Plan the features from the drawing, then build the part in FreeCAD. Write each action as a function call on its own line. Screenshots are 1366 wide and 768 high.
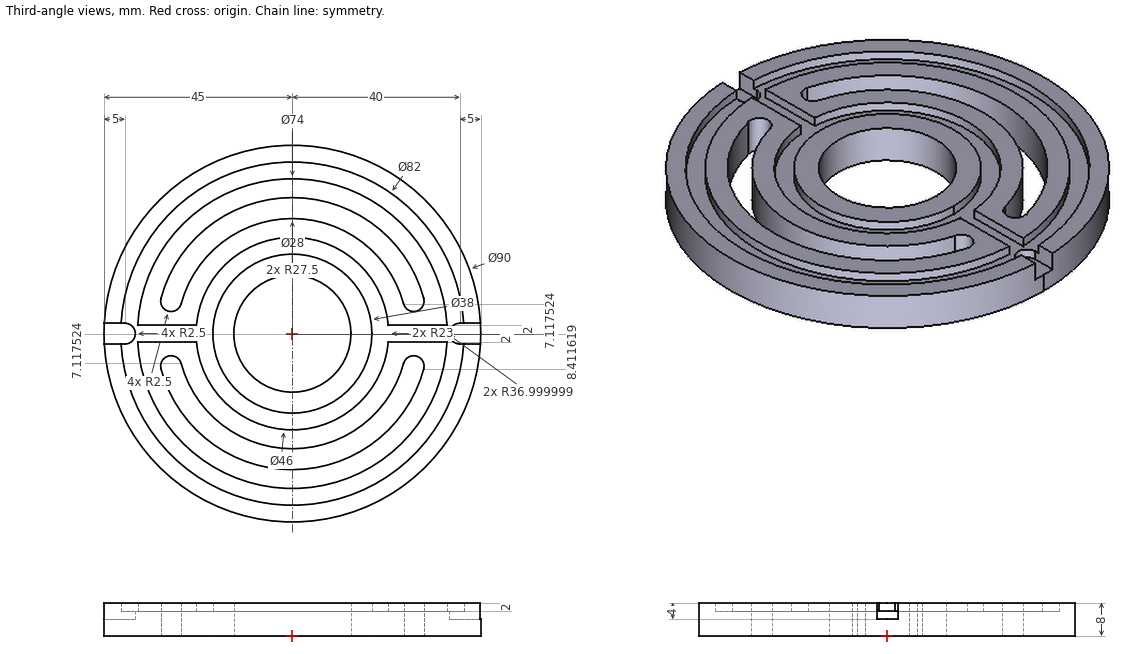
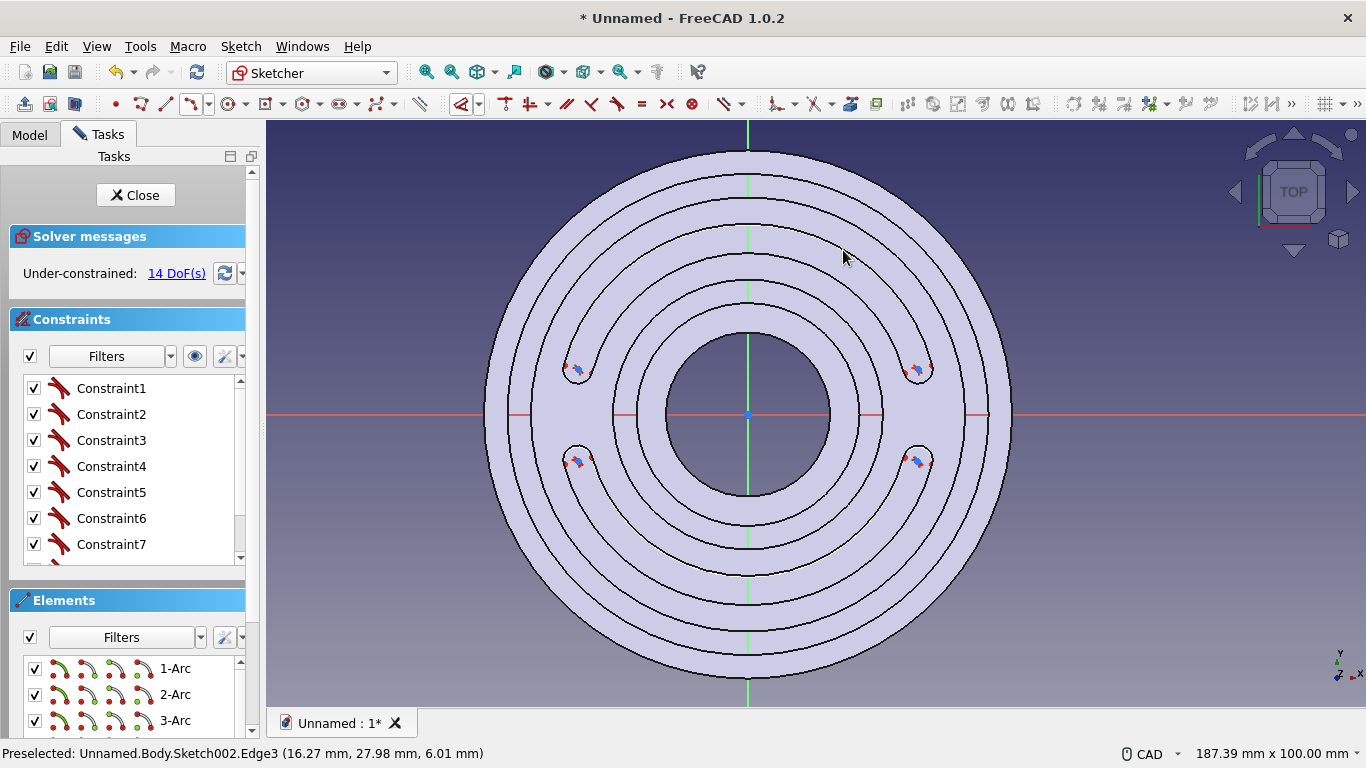
click(829, 275)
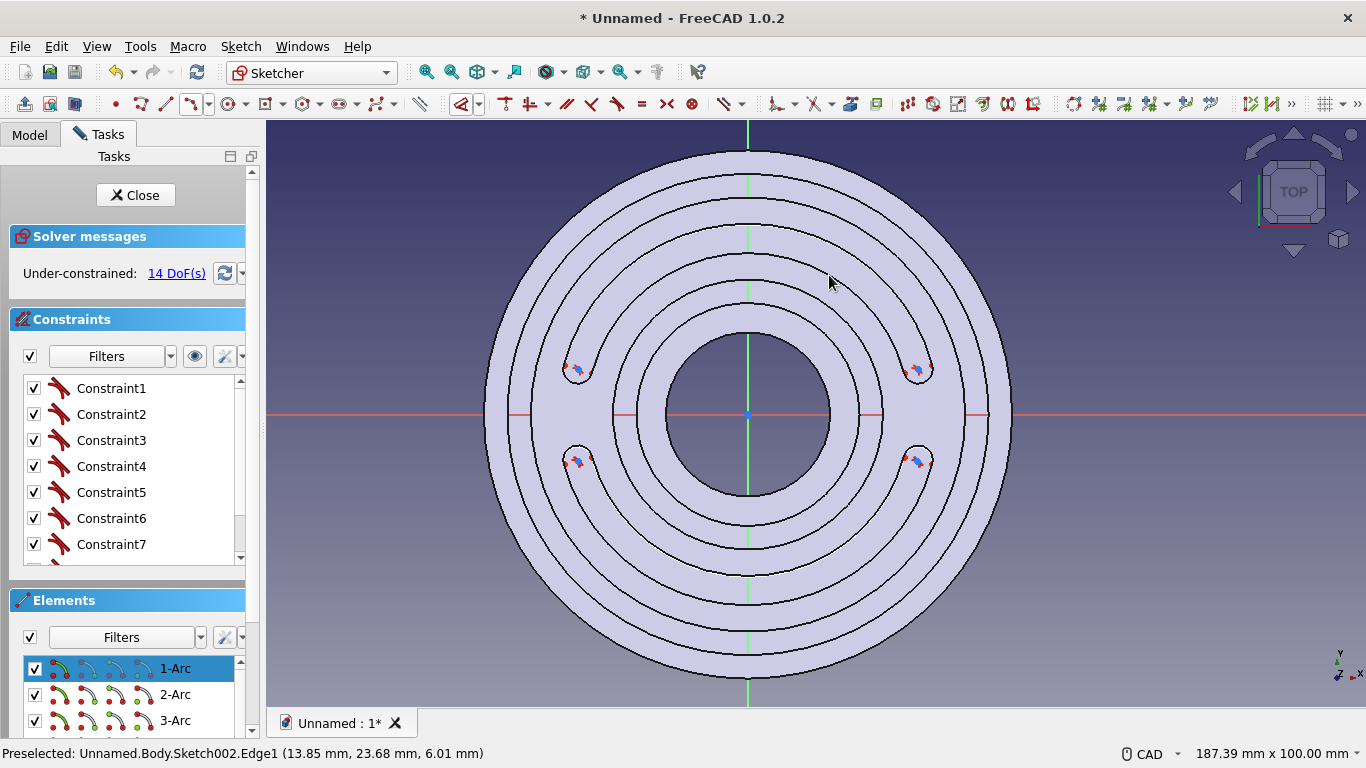
click(653, 581)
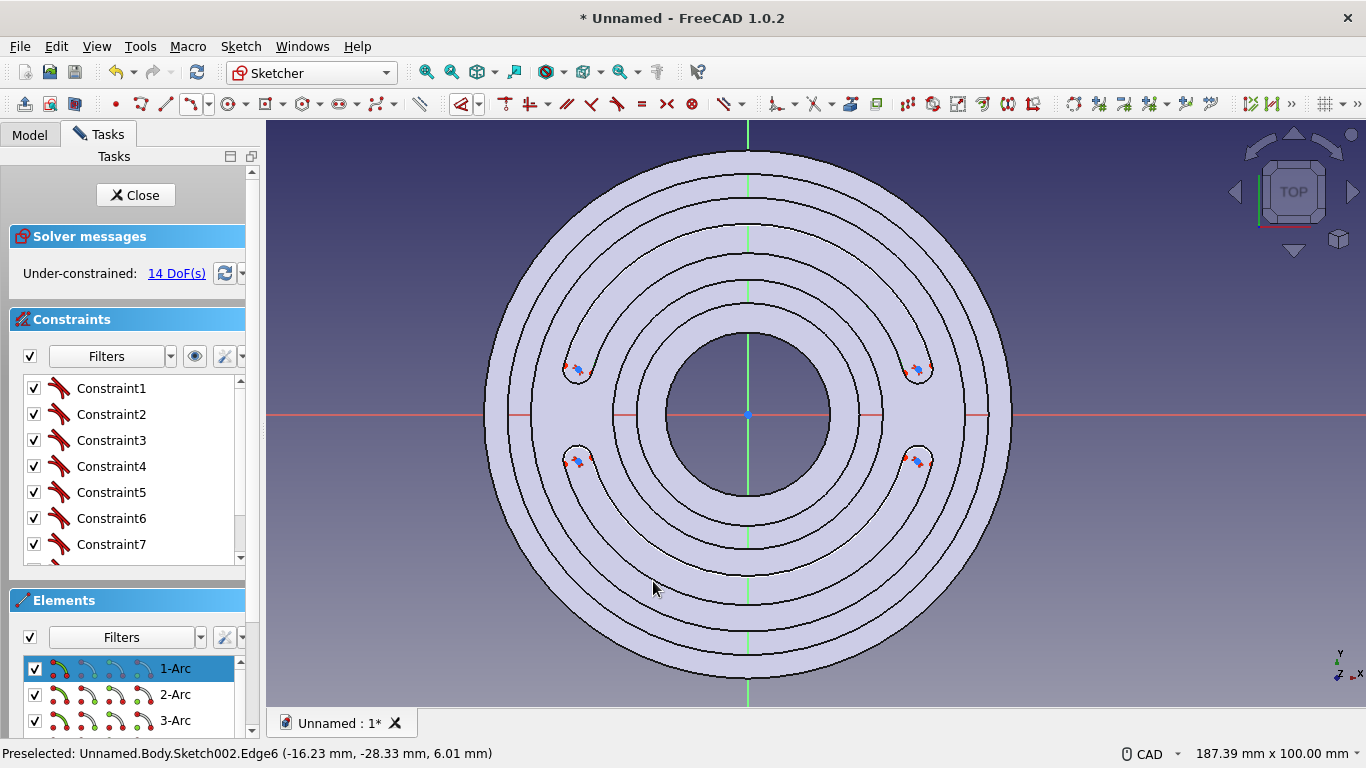
key(c)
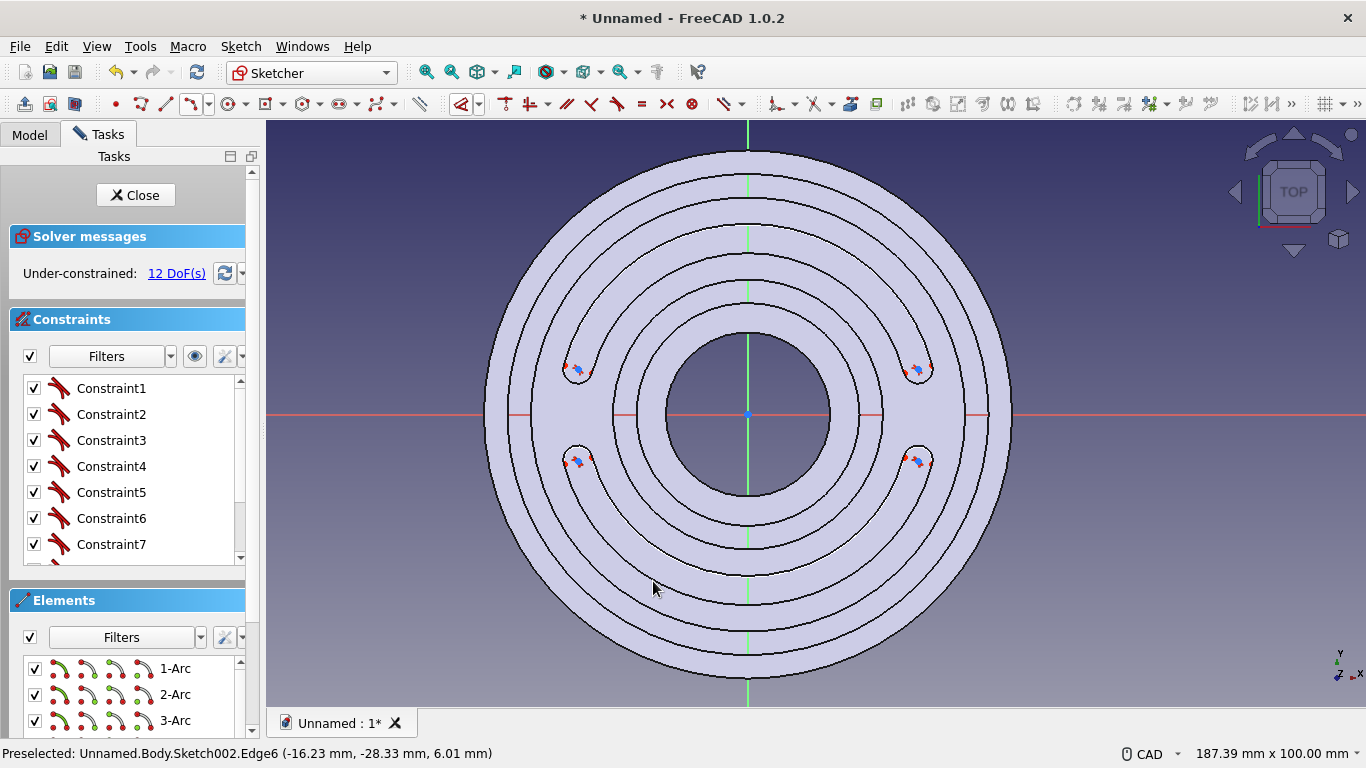
click(829, 275)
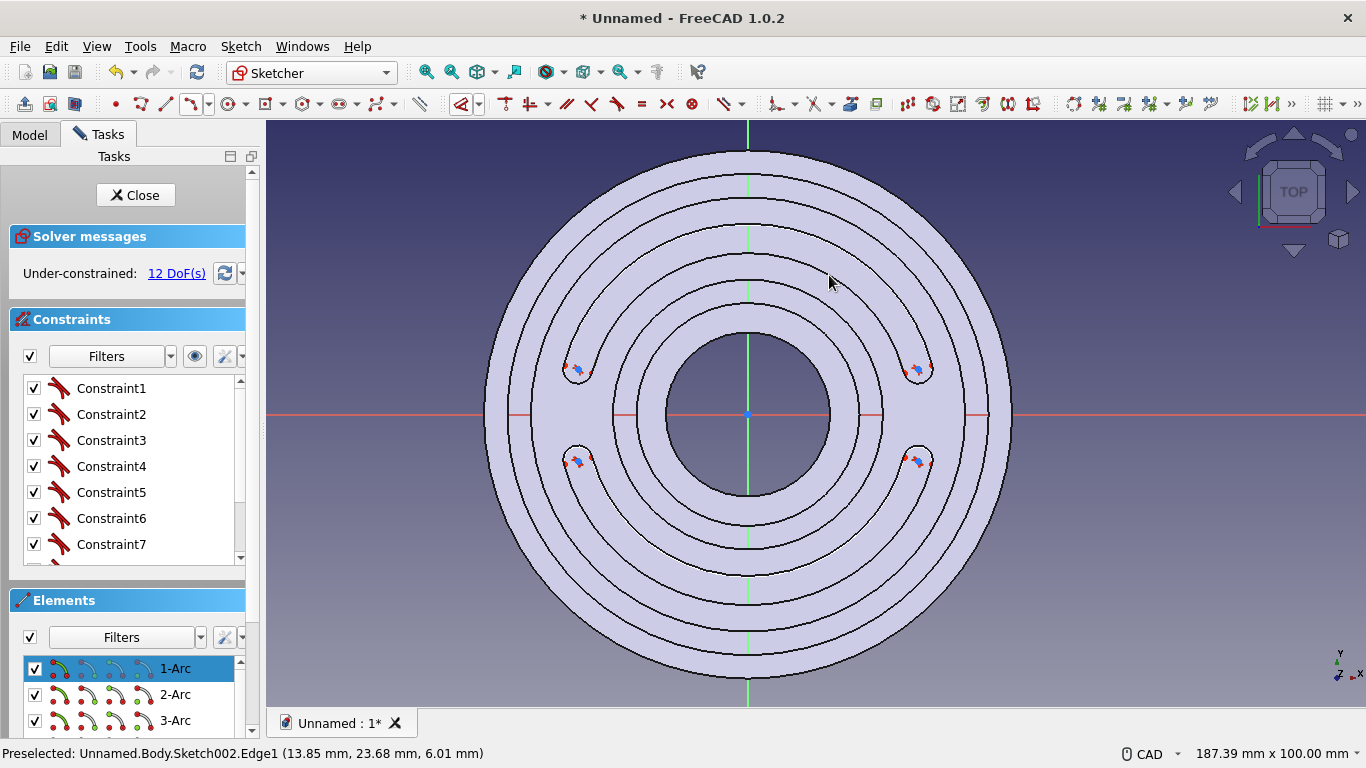
click(667, 555)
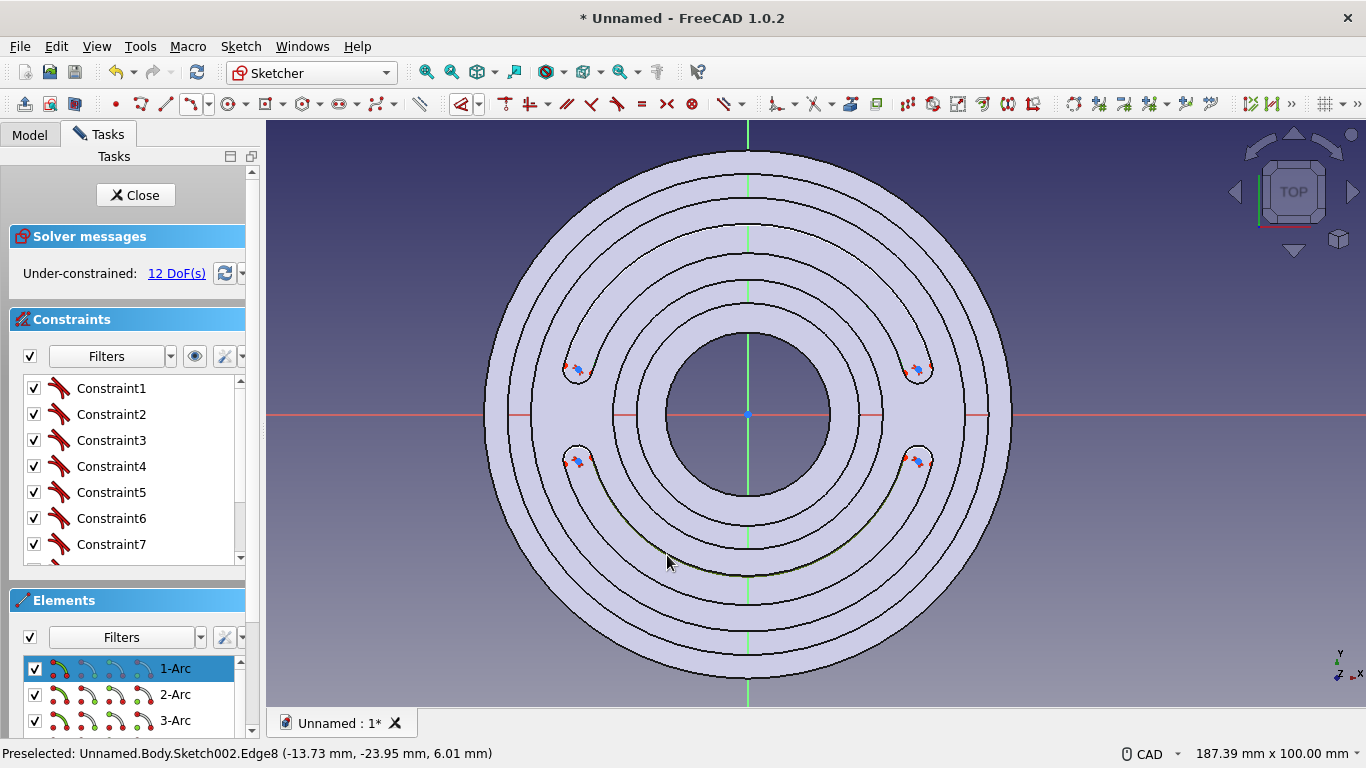
key(c)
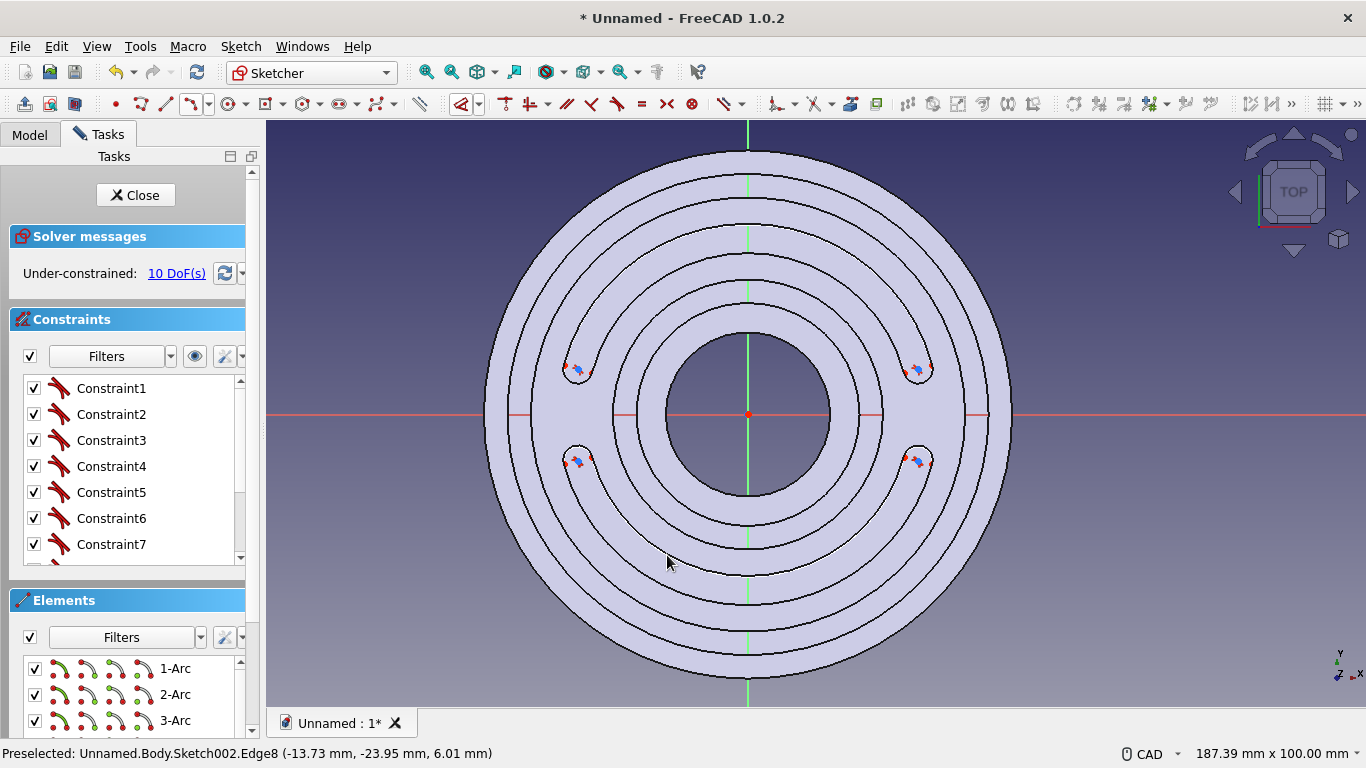
scroll(748, 415, up, 6)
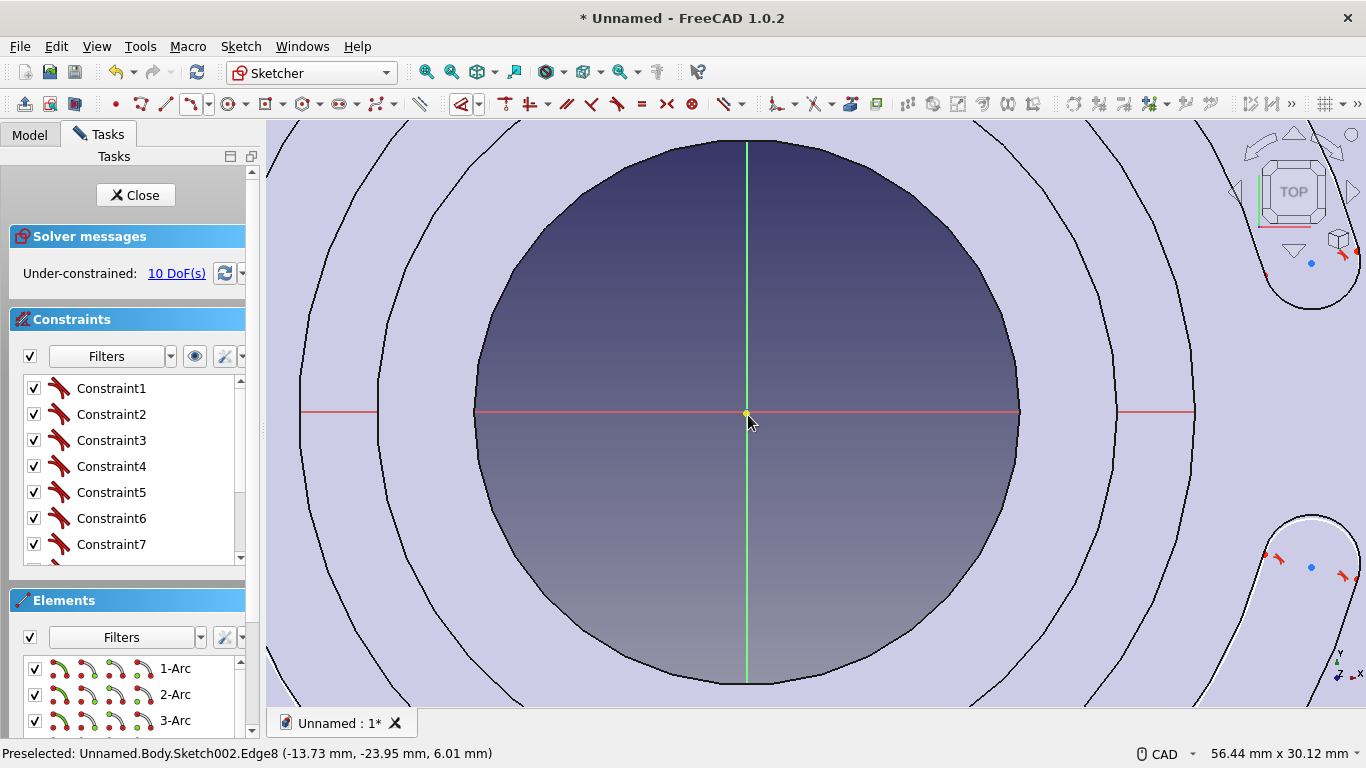
drag(737, 402, 757, 424)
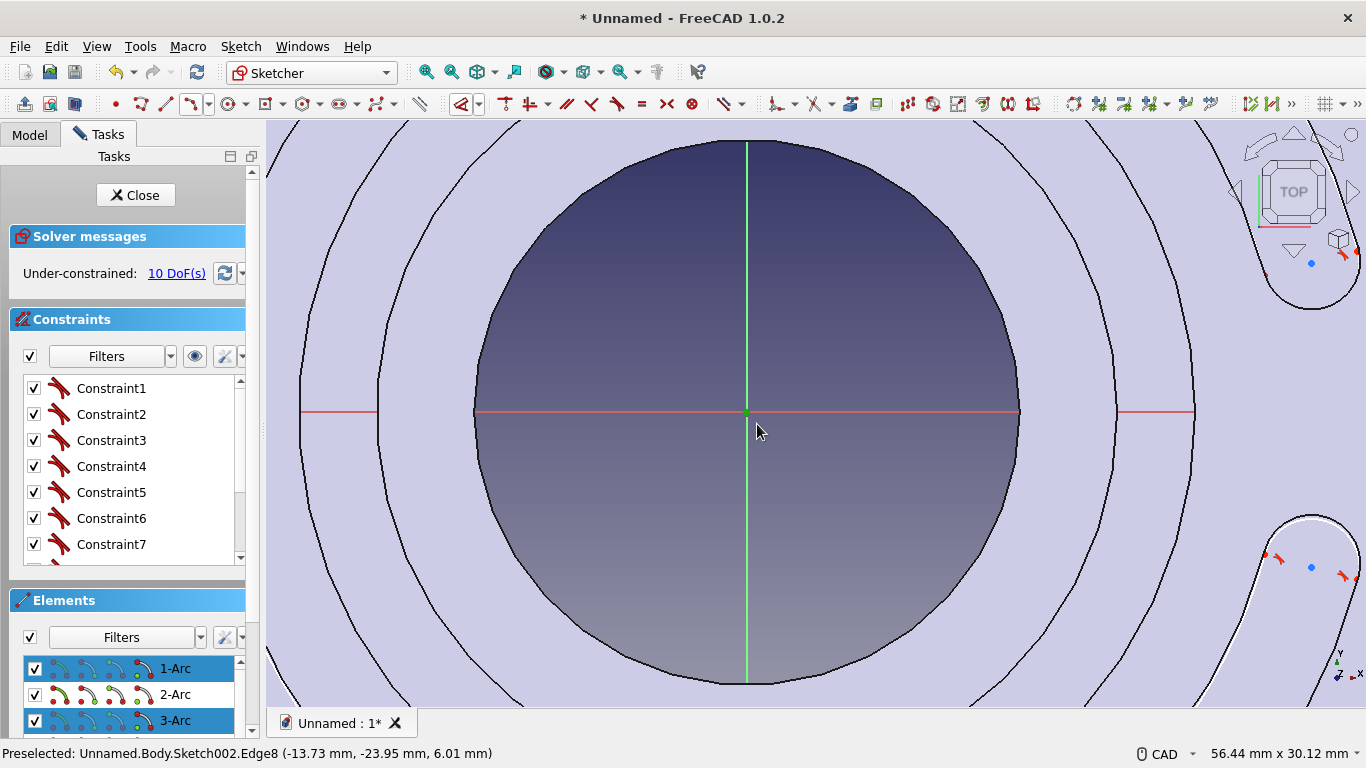
click(505, 104)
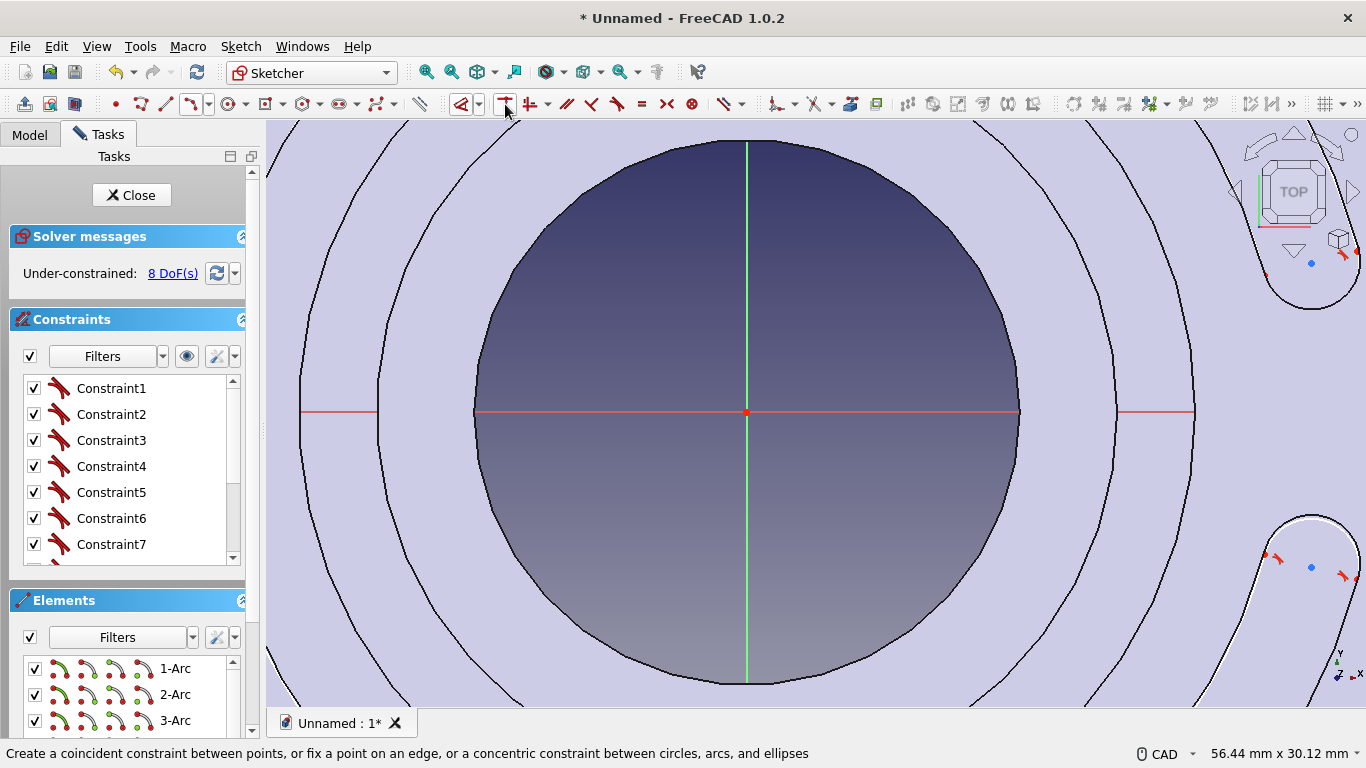
scroll(748, 414, down, 6)